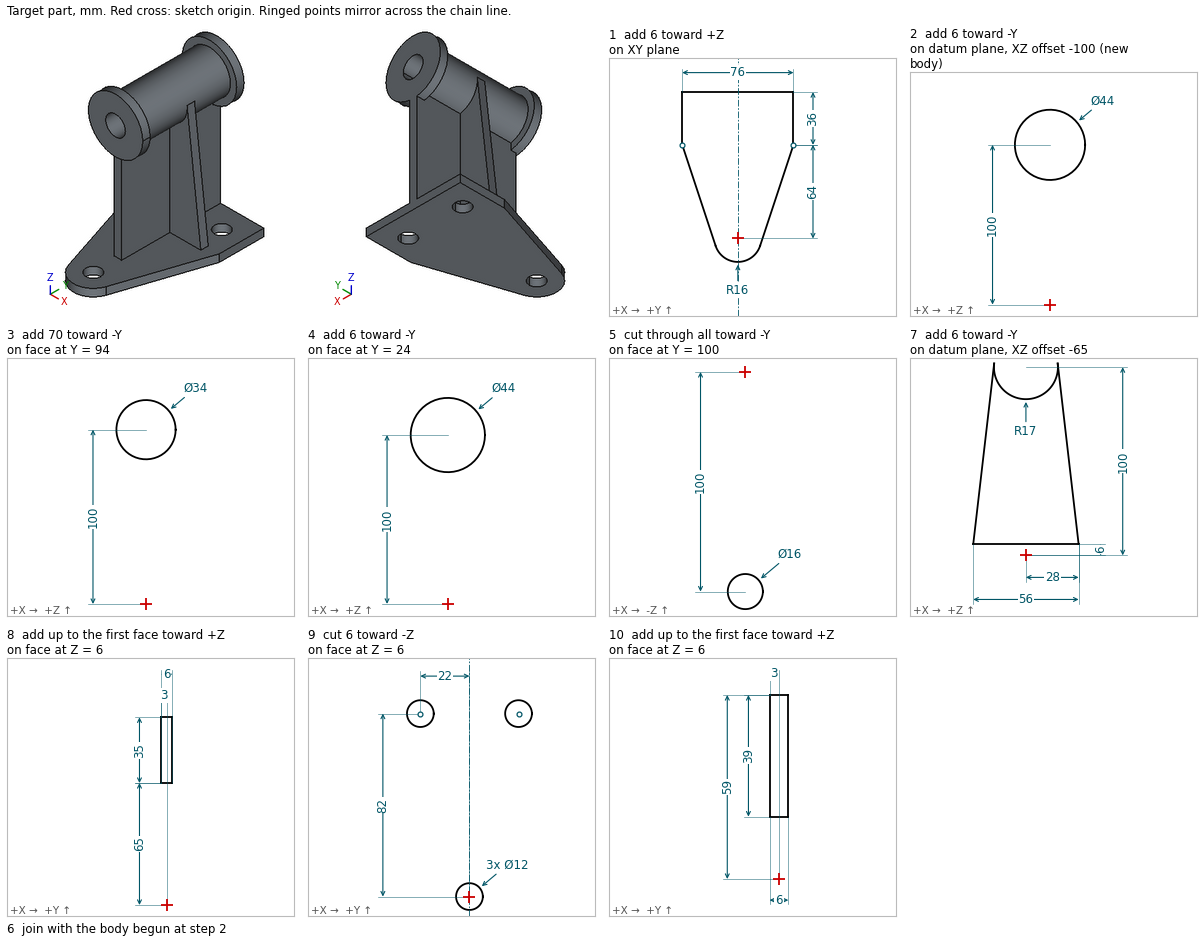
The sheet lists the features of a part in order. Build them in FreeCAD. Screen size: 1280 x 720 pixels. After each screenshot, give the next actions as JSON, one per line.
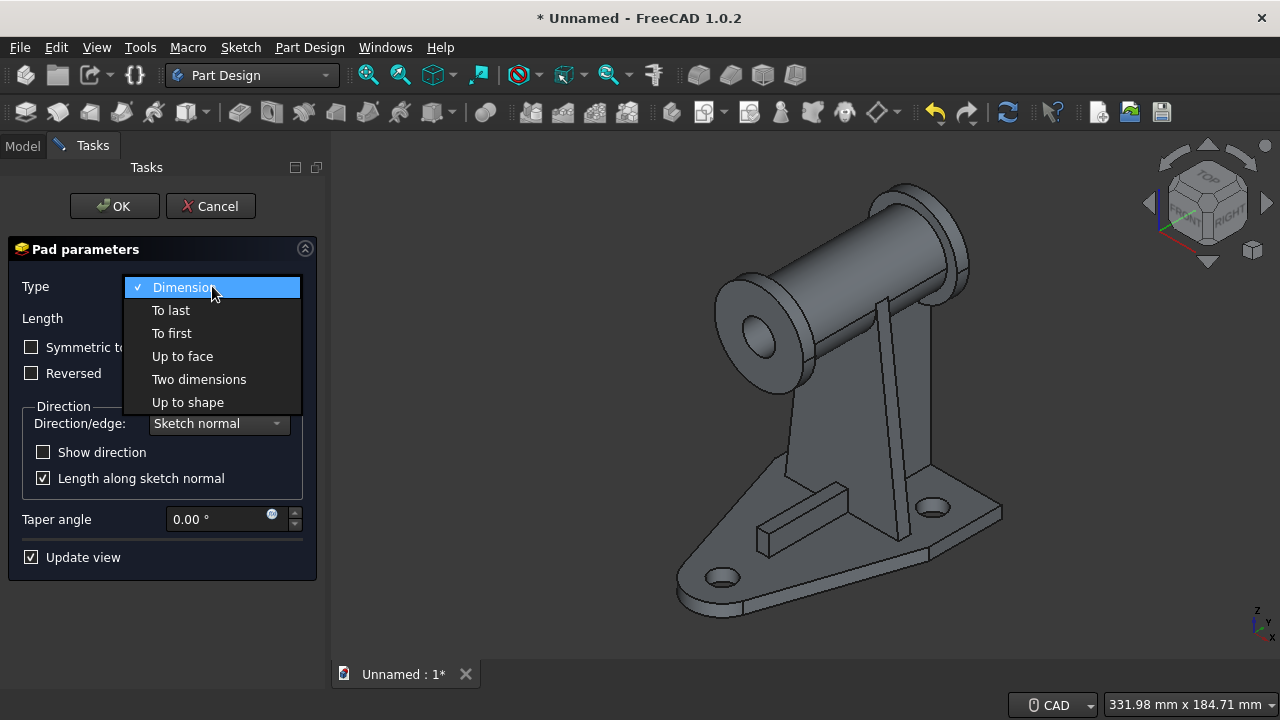
{"action": "left_click", "coordinate": [212, 334]}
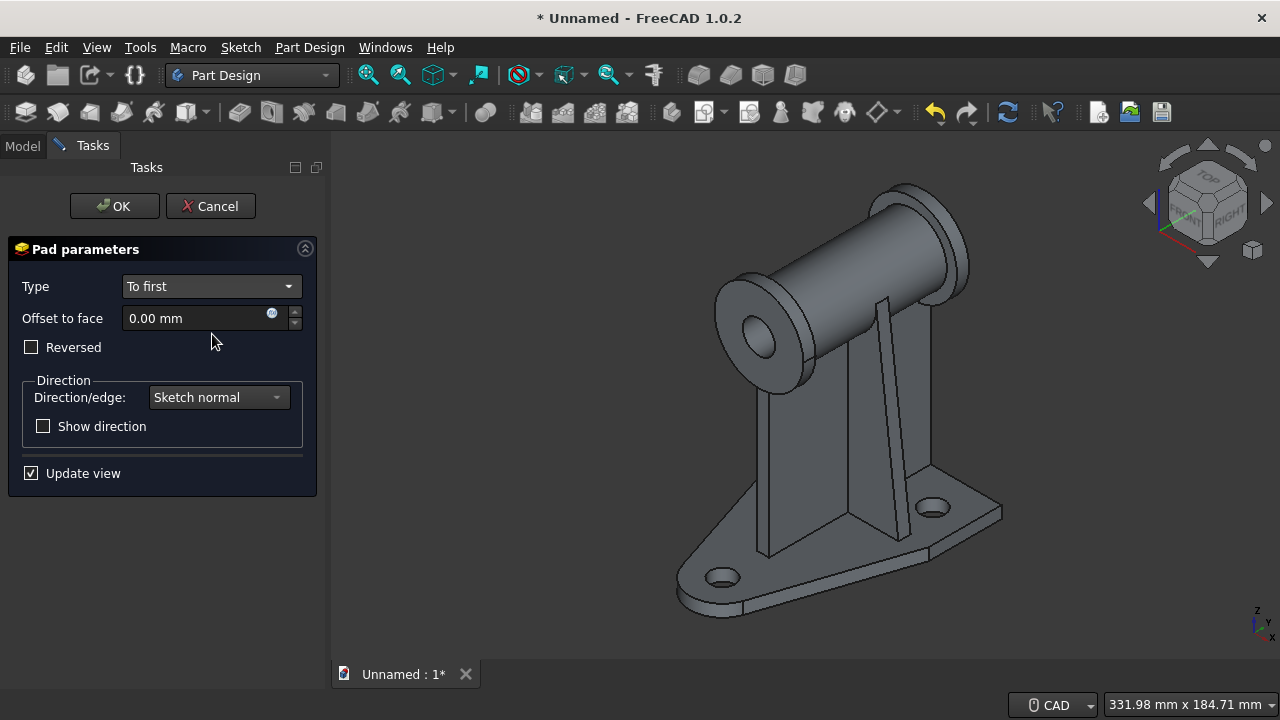
{"action": "left_click", "coordinate": [115, 206]}